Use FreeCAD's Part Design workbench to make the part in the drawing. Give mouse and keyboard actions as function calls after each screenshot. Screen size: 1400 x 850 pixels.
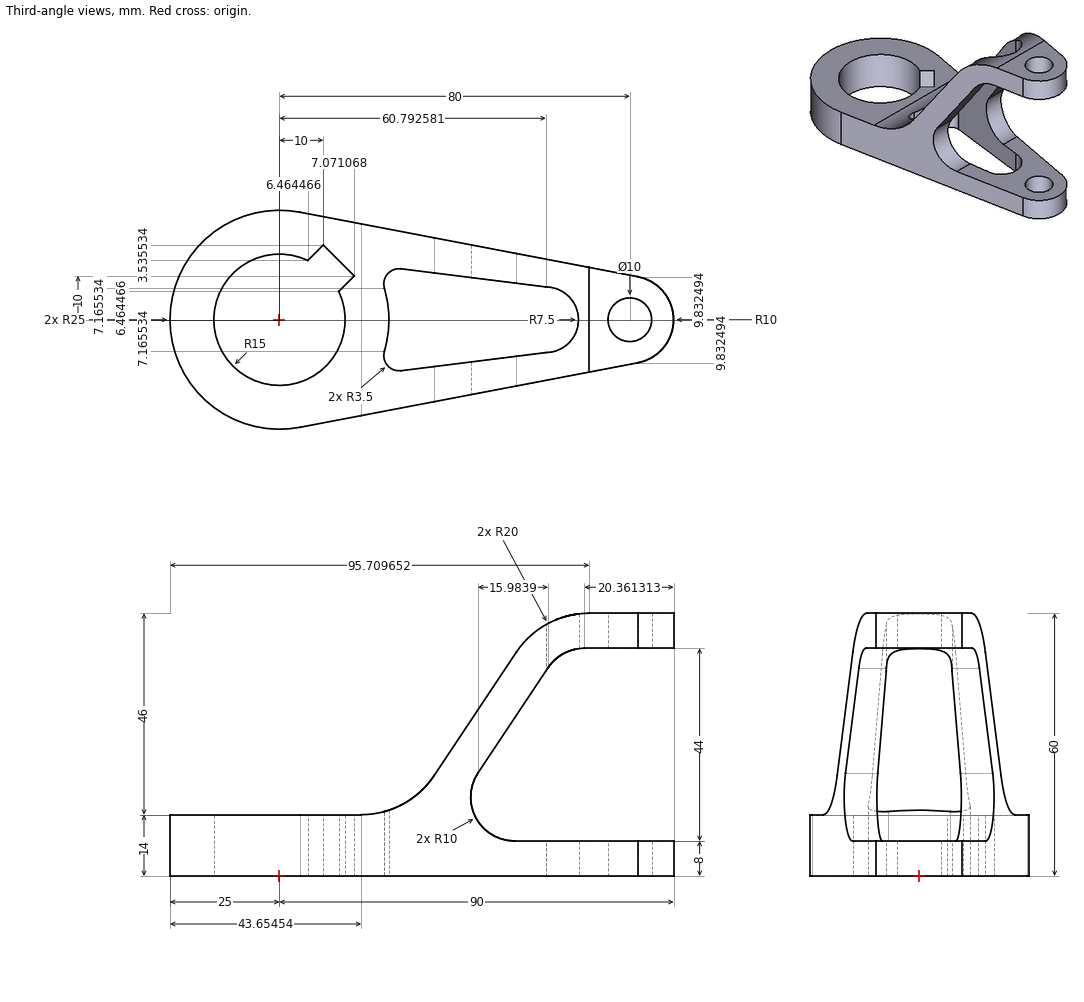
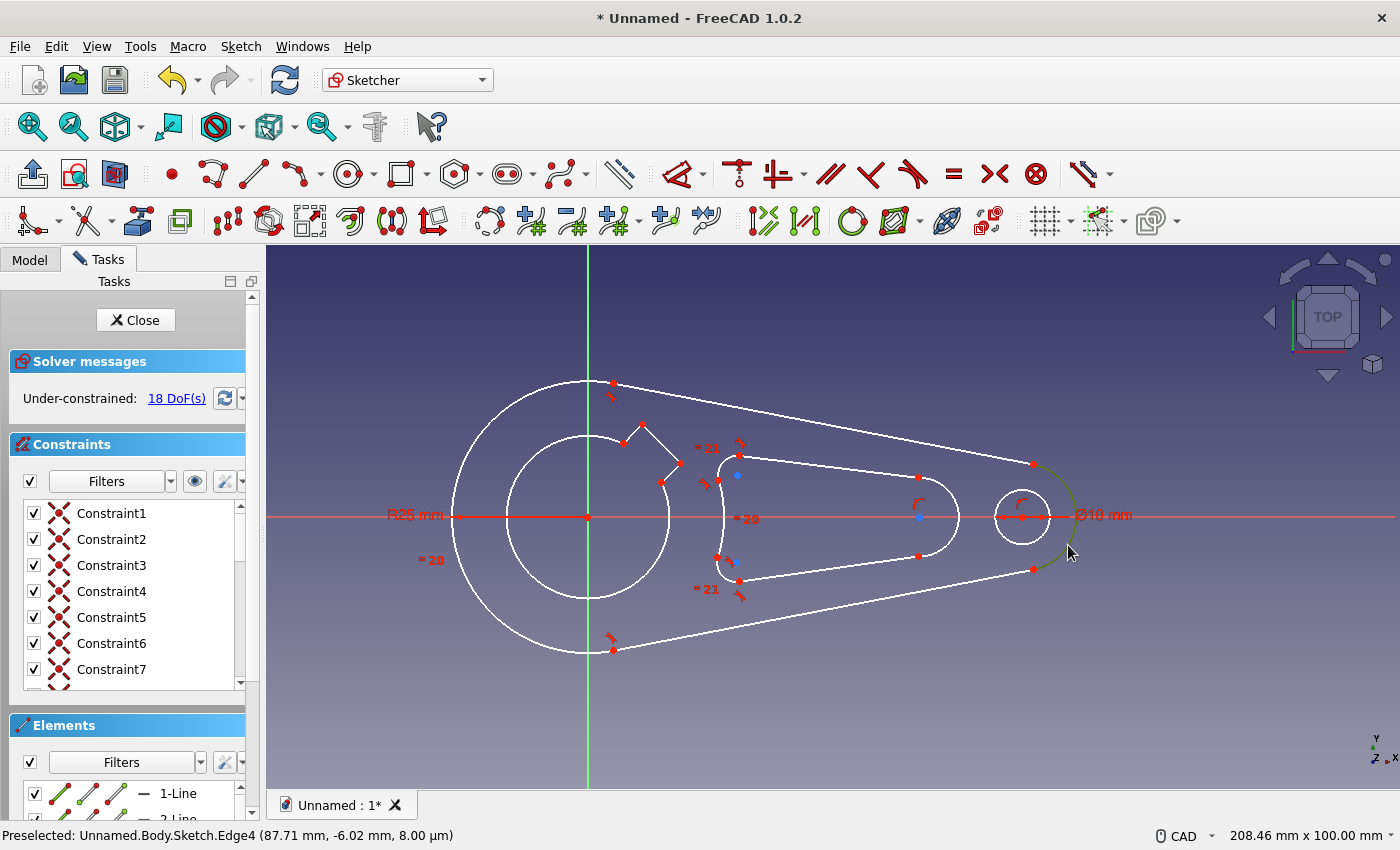
key(k)
key(r)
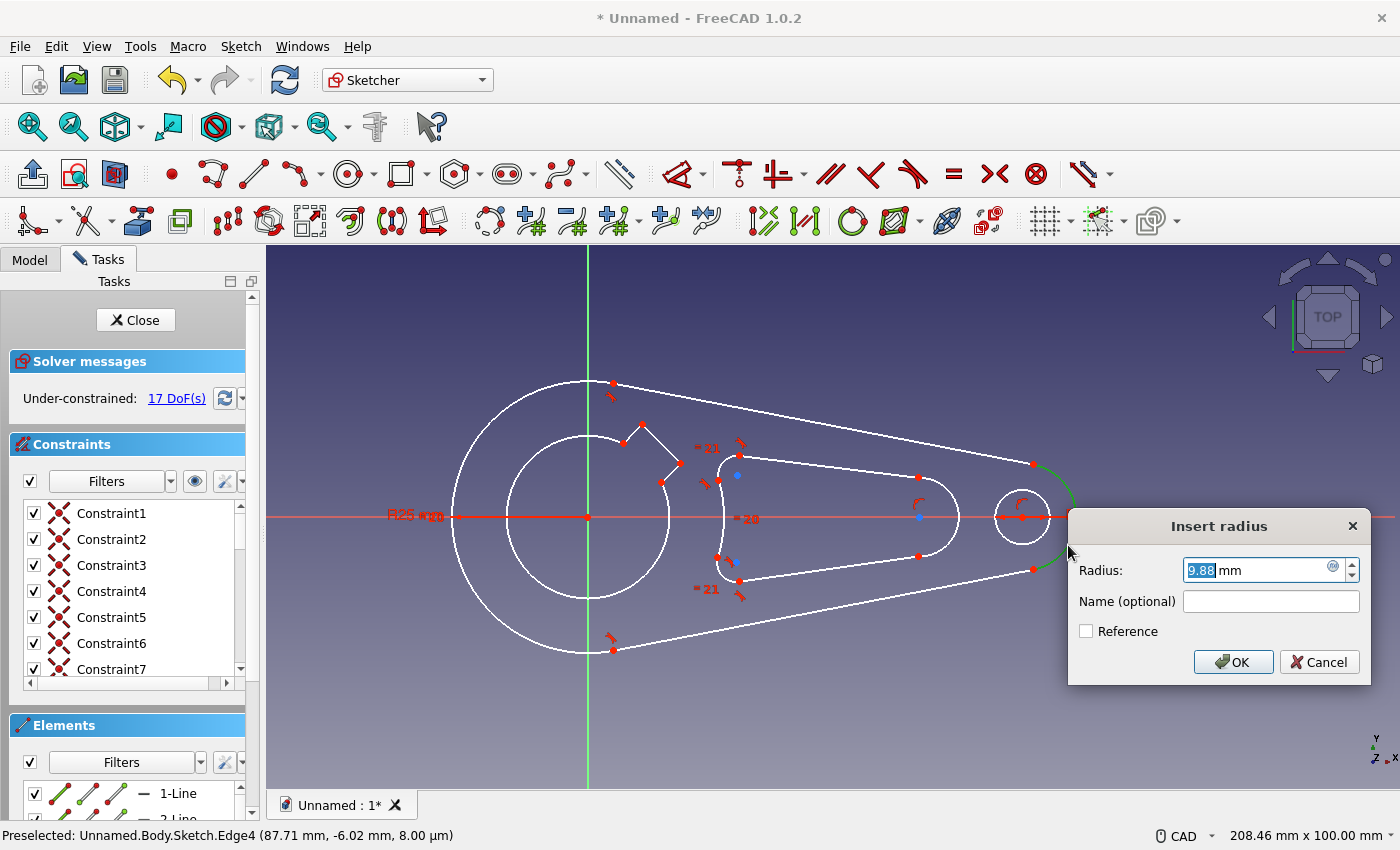
text(10)
key(Return)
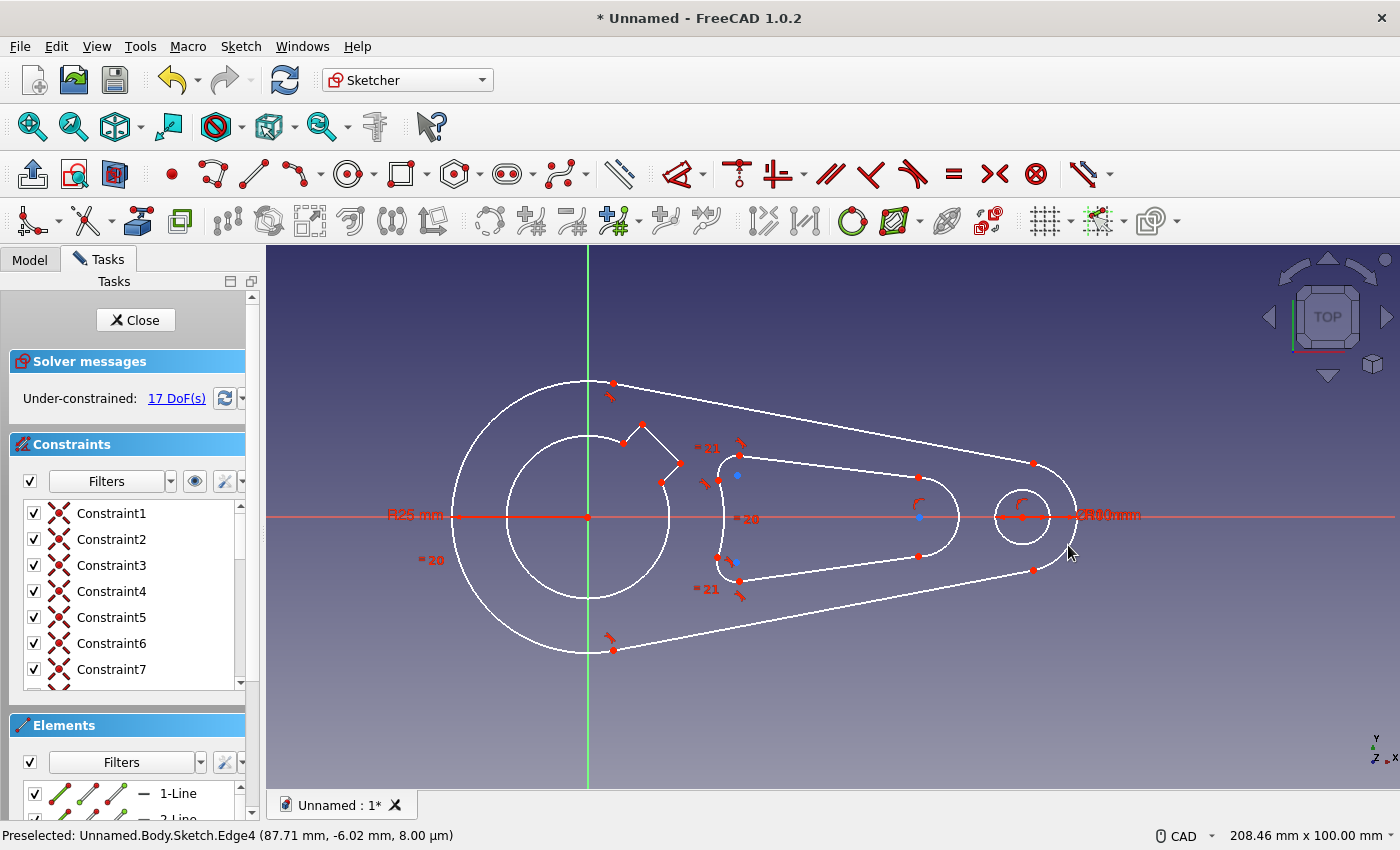
click(951, 541)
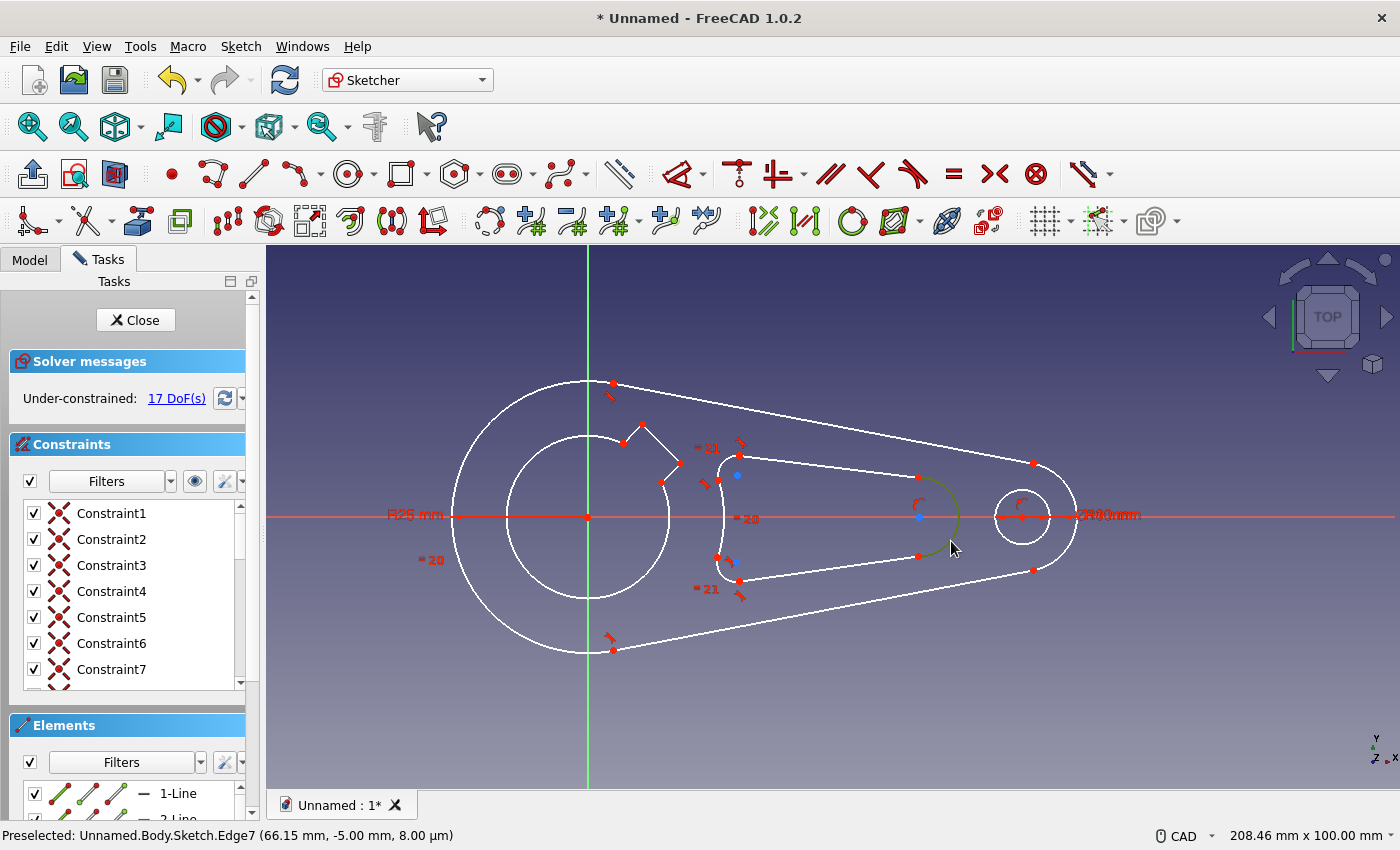
click(702, 174)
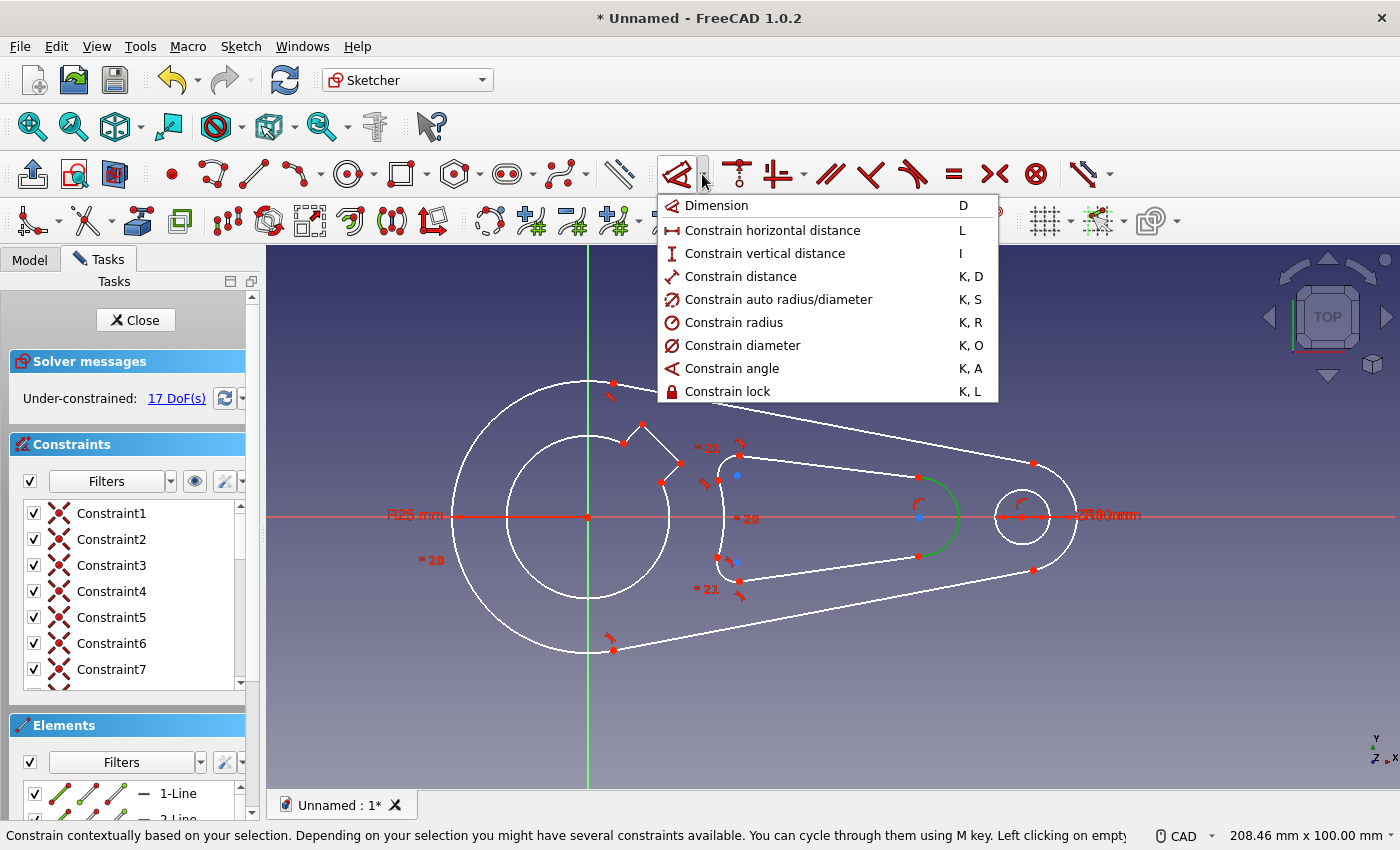
click(828, 322)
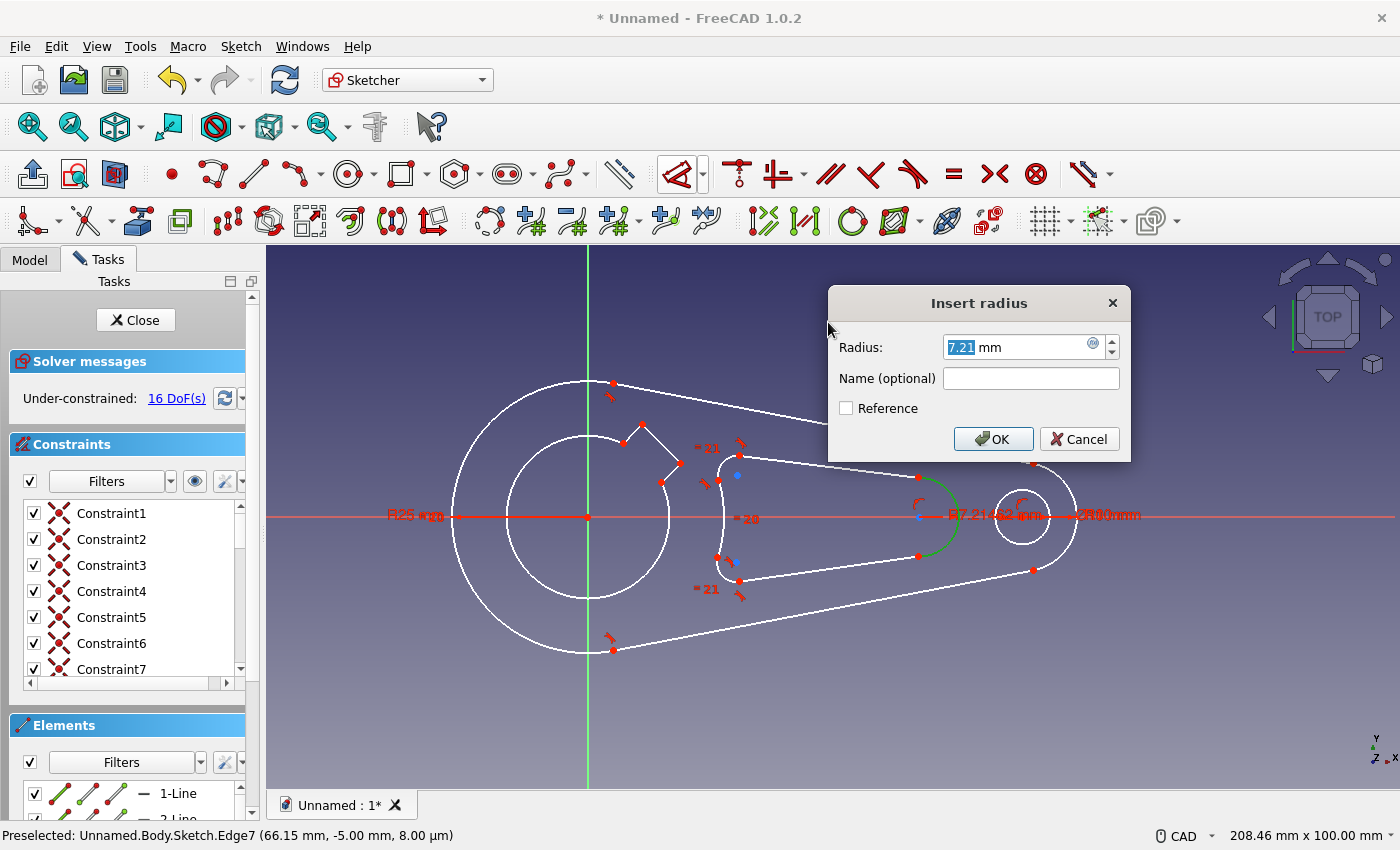
text(7.5)
key(Return)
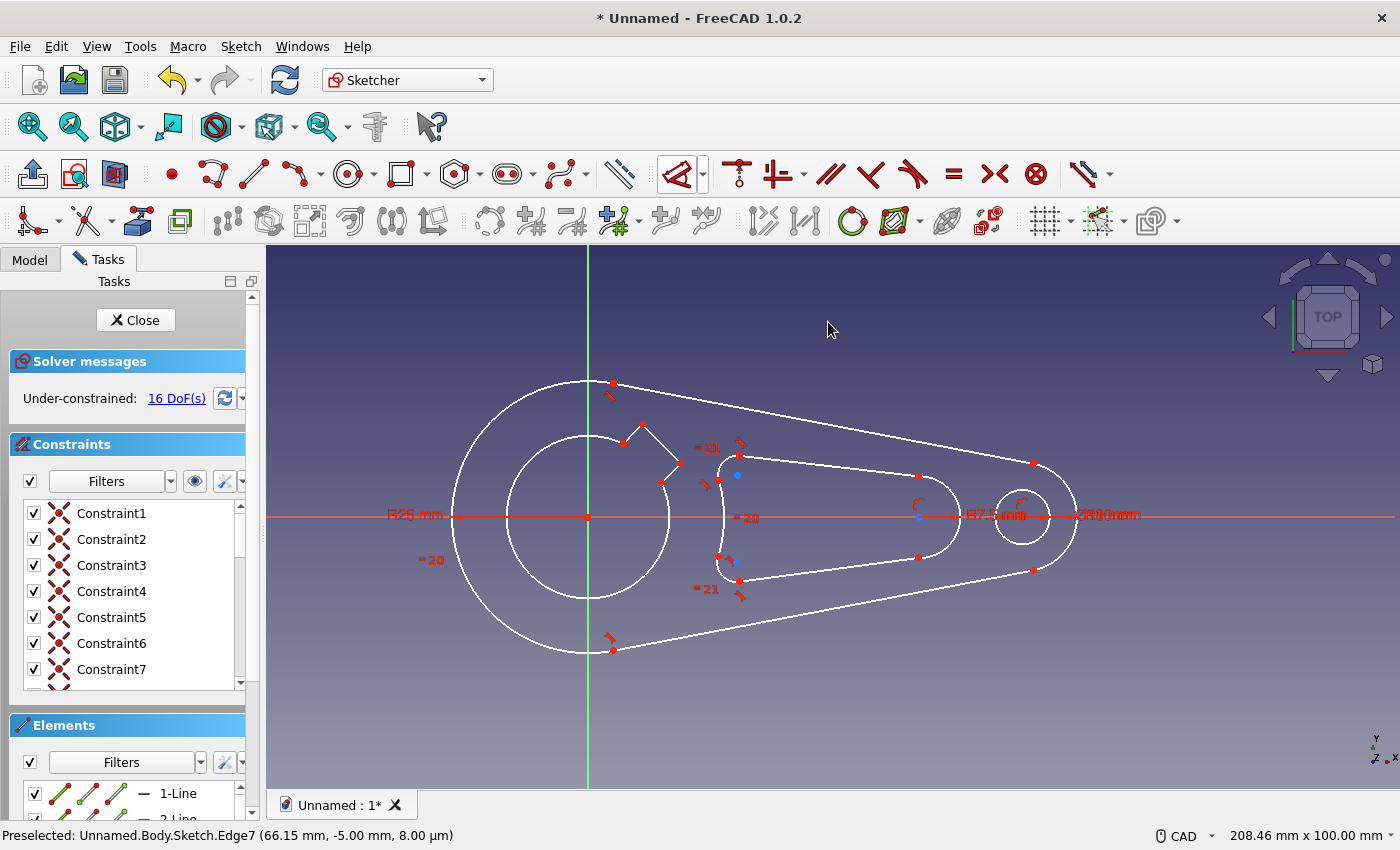
scroll(718, 568, up, 4)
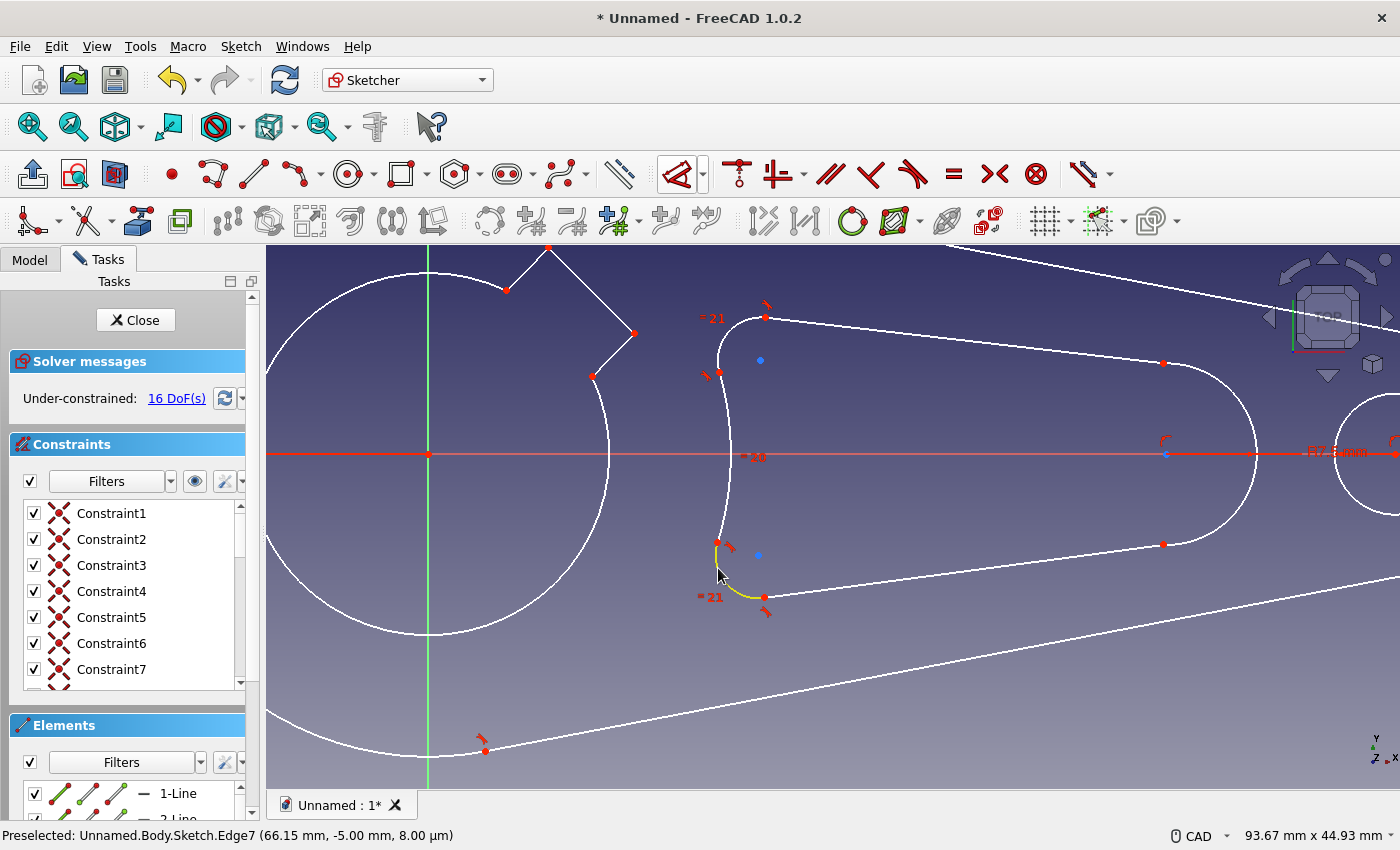
click(718, 568)